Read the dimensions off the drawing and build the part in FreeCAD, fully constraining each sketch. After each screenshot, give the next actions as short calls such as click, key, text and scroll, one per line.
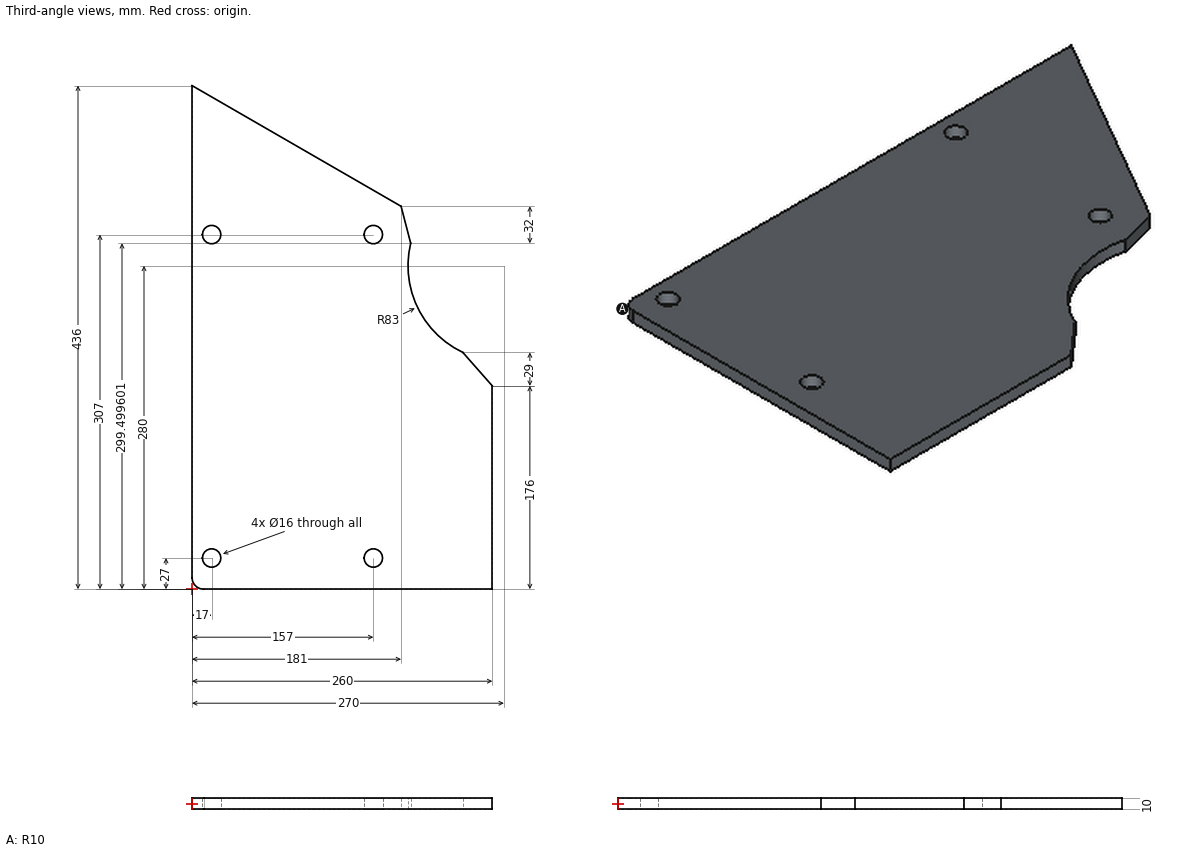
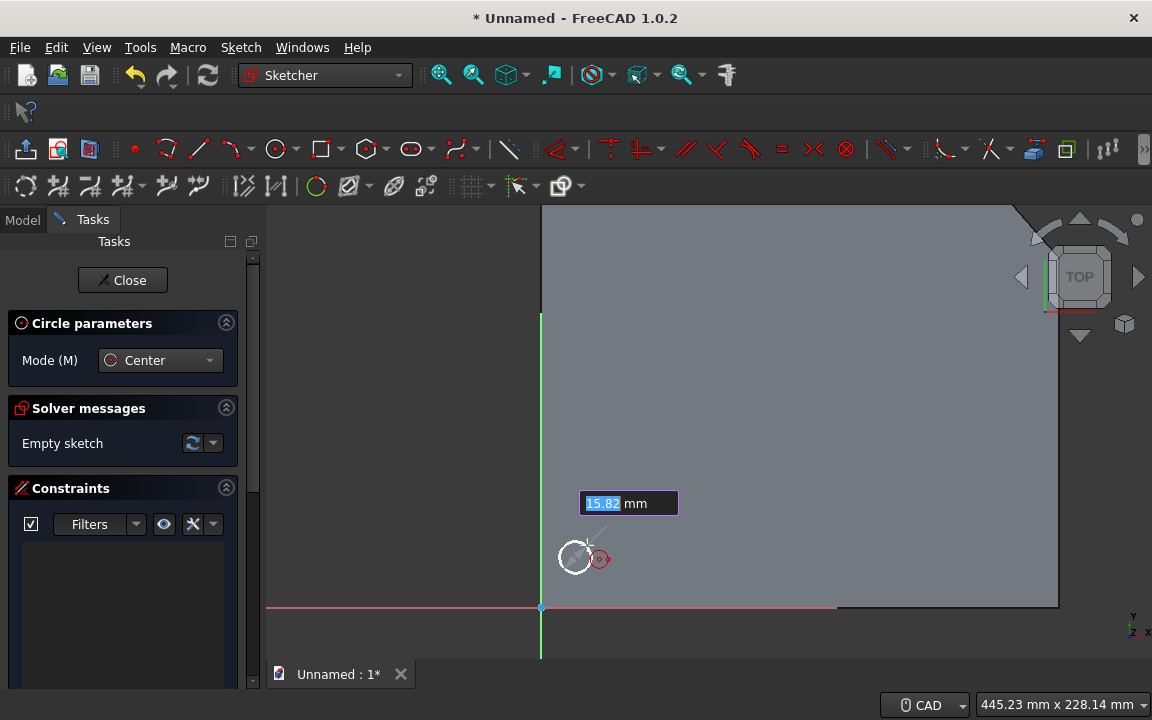
click(587, 543)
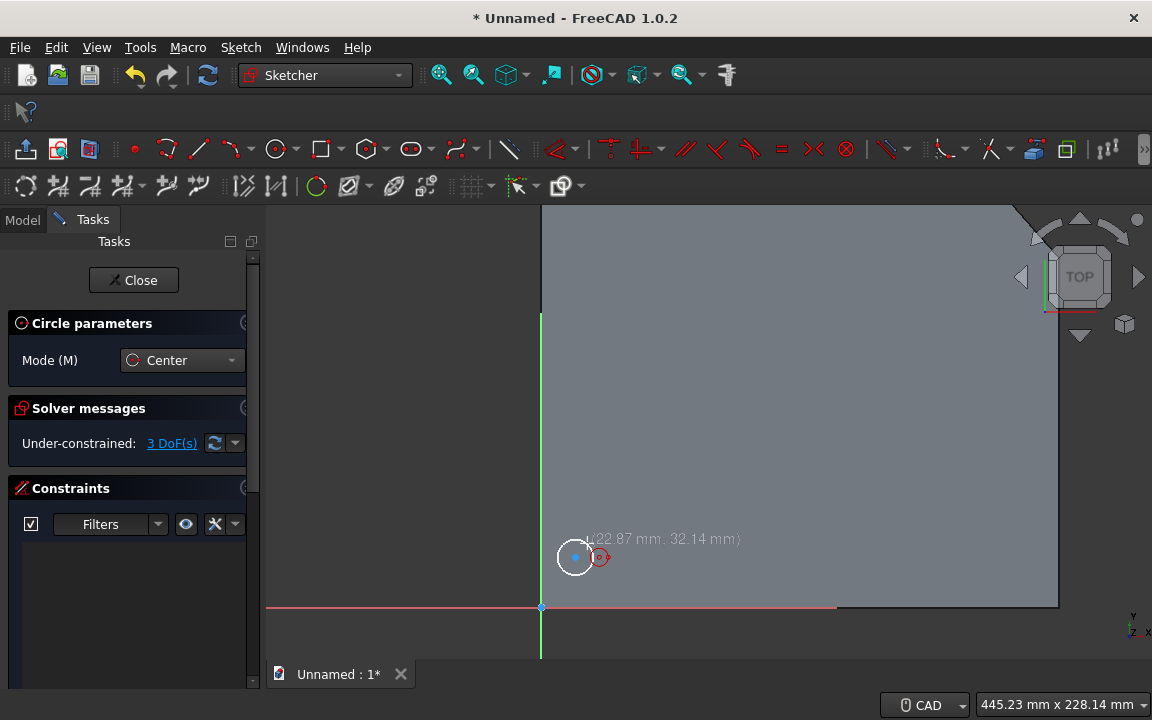
scroll(854, 554, up, 2)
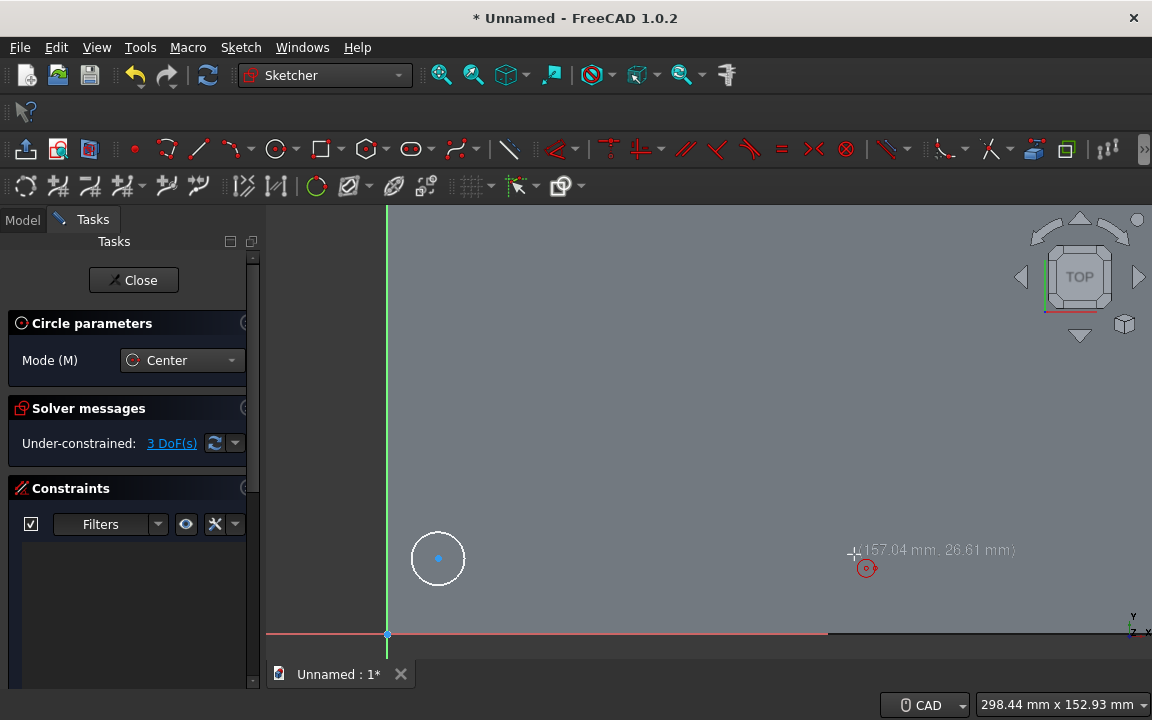
scroll(644, 546, down, 6)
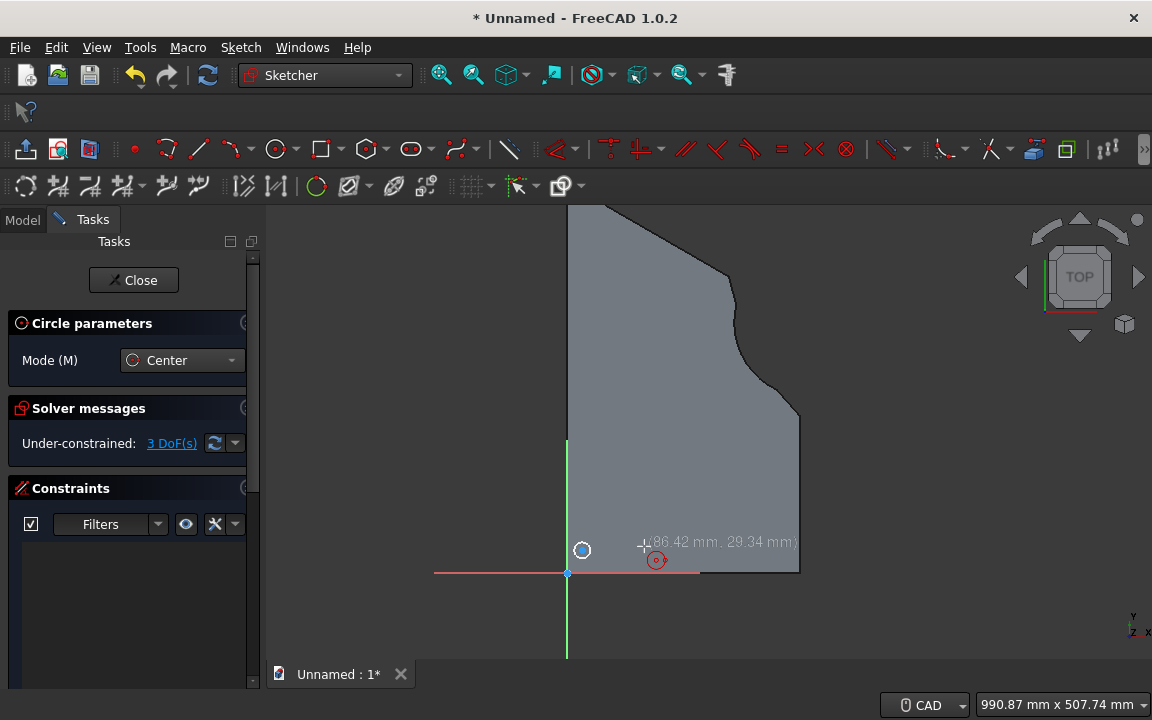
click(707, 549)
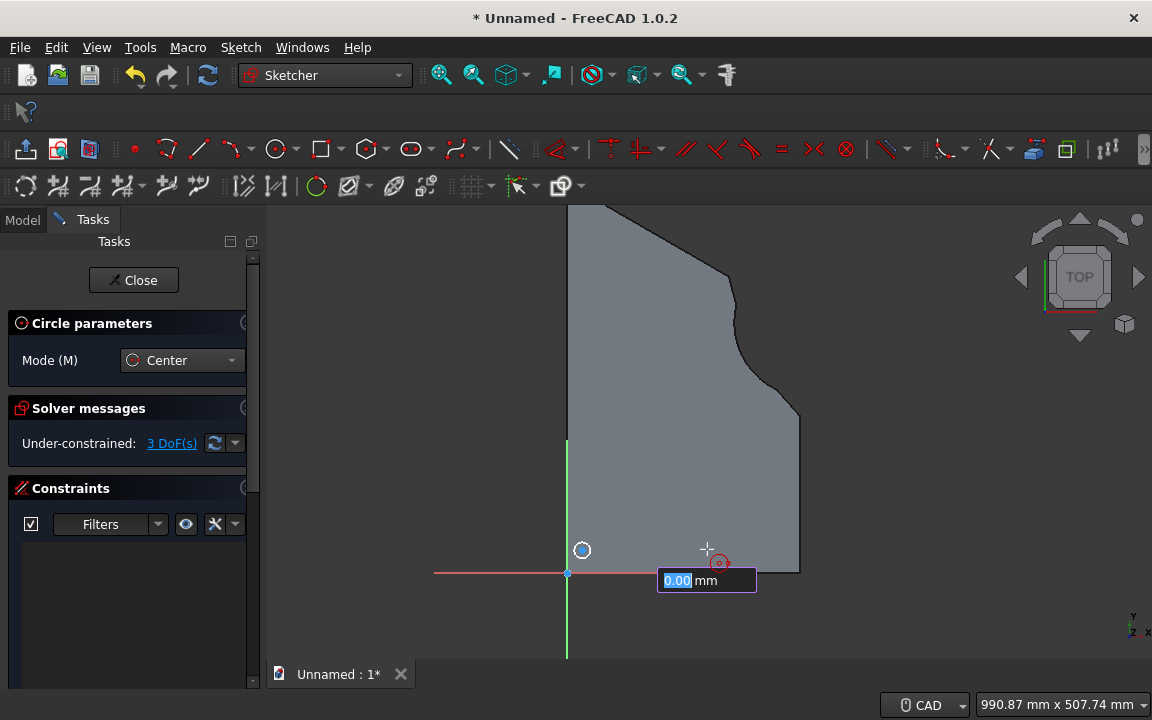
scroll(712, 544, up, 4)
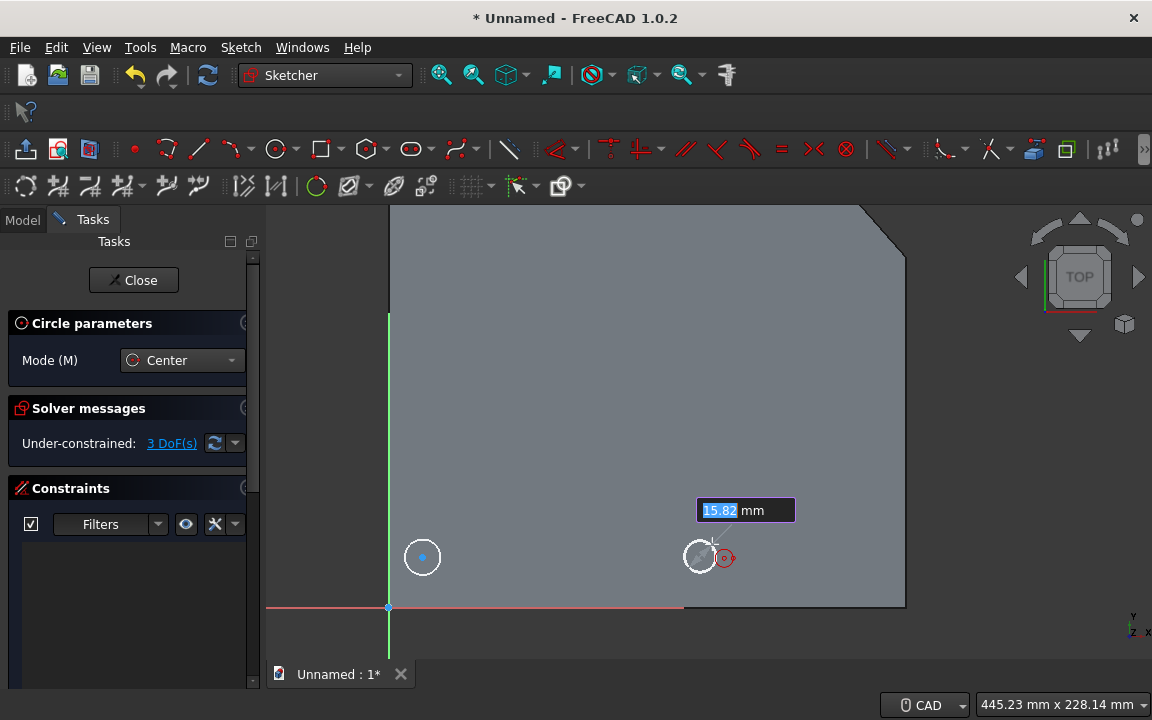
click(712, 543)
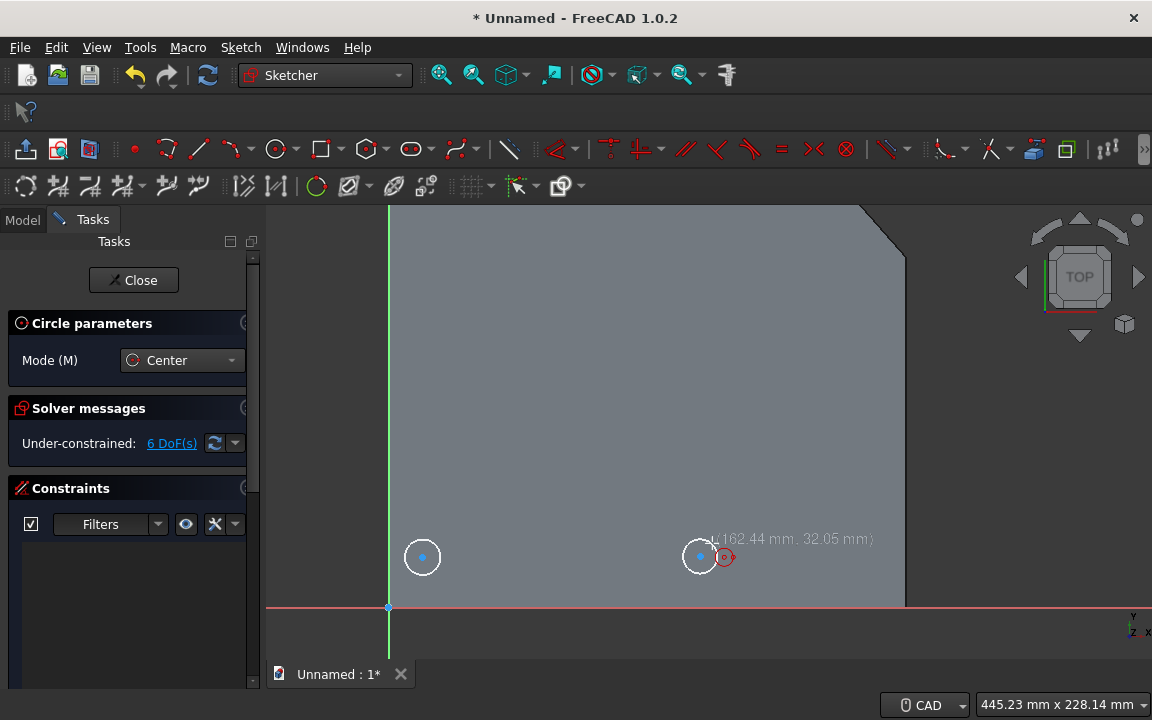
scroll(712, 544, down, 4)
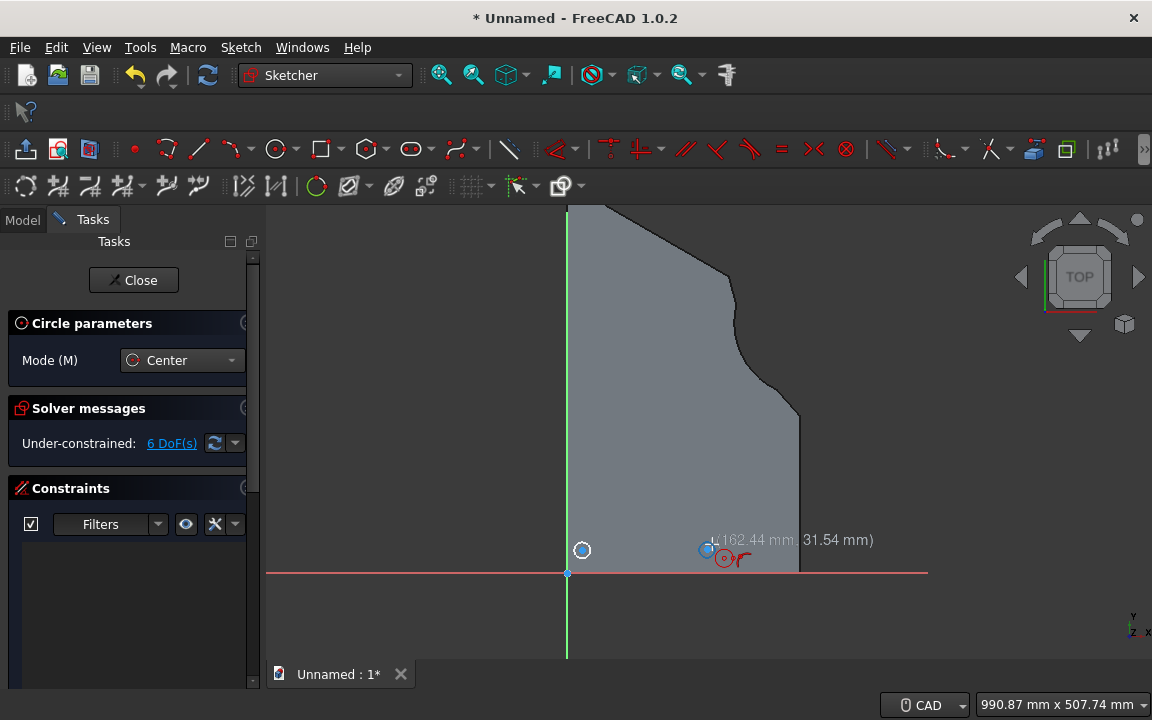
scroll(707, 299, up, 6)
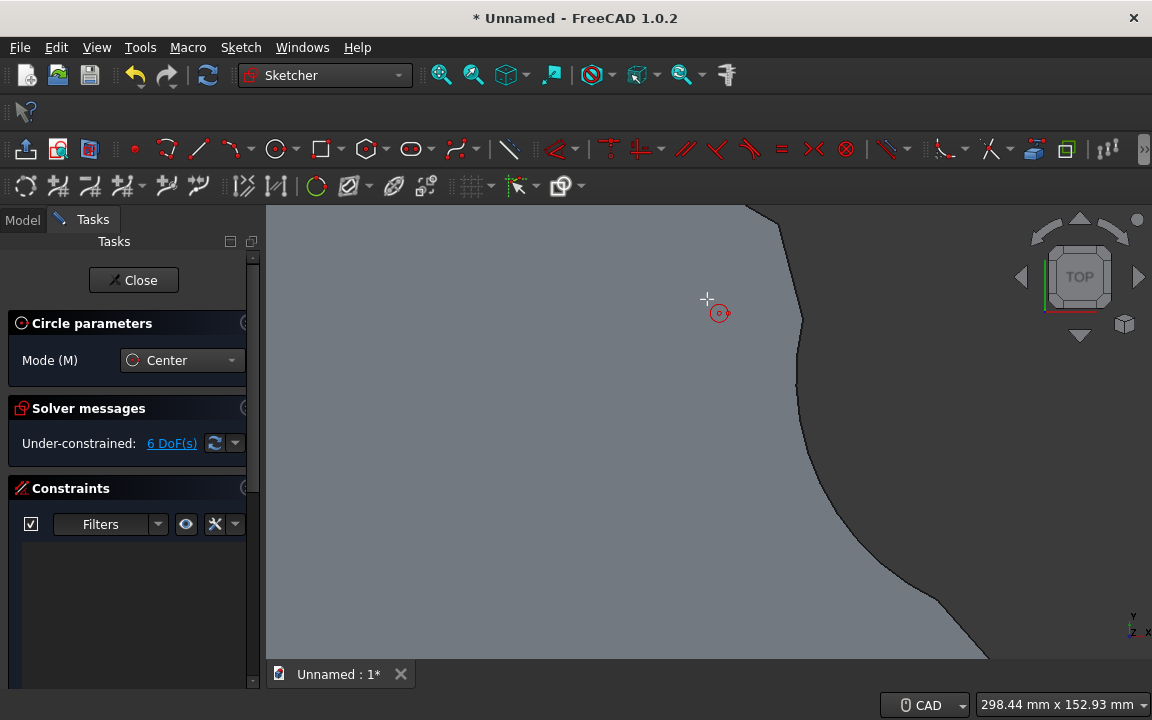
scroll(707, 299, down, 6)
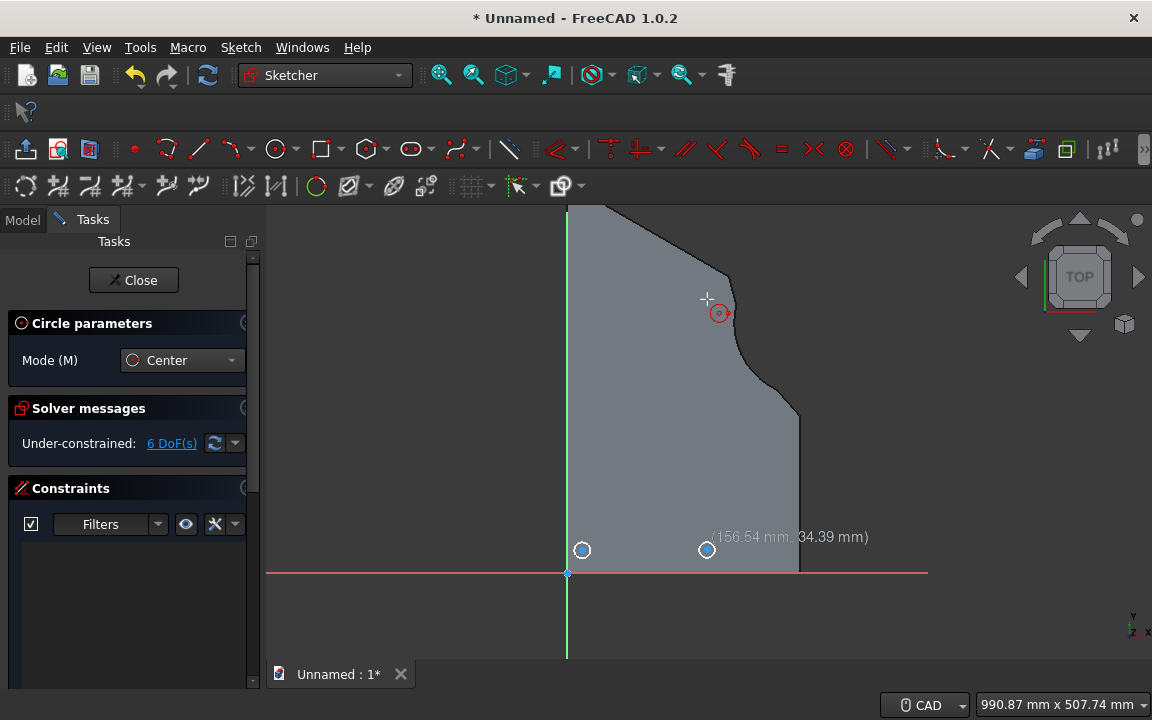
click(707, 299)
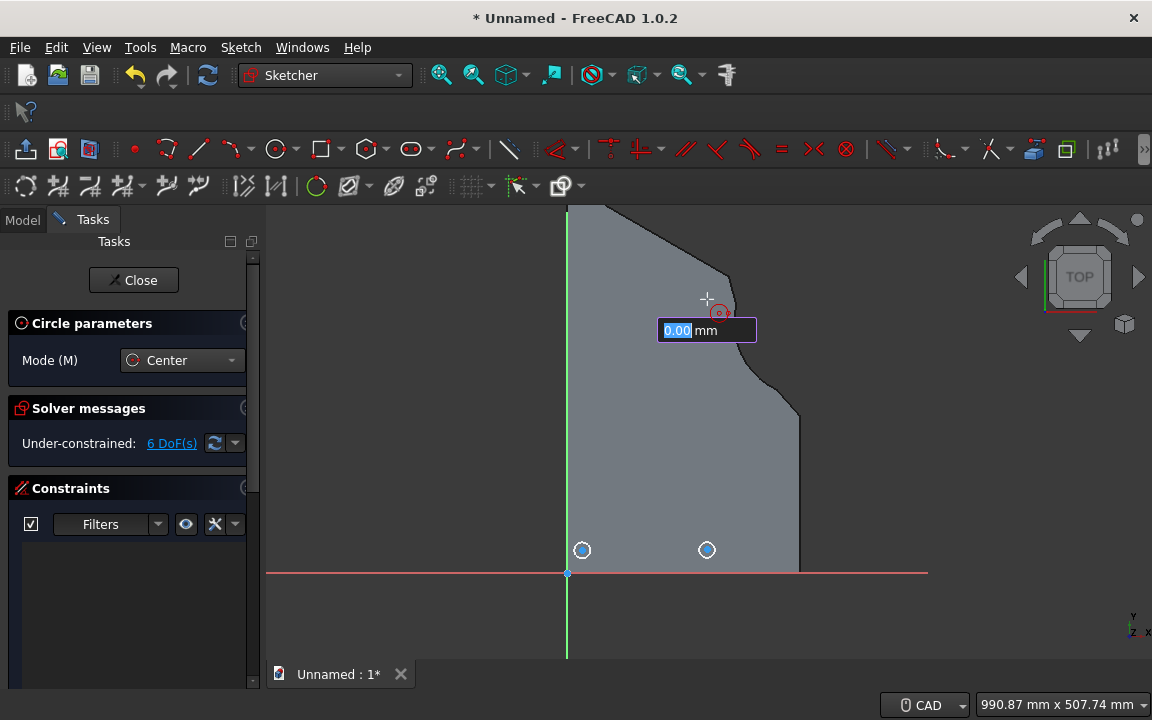
scroll(712, 293, up, 4)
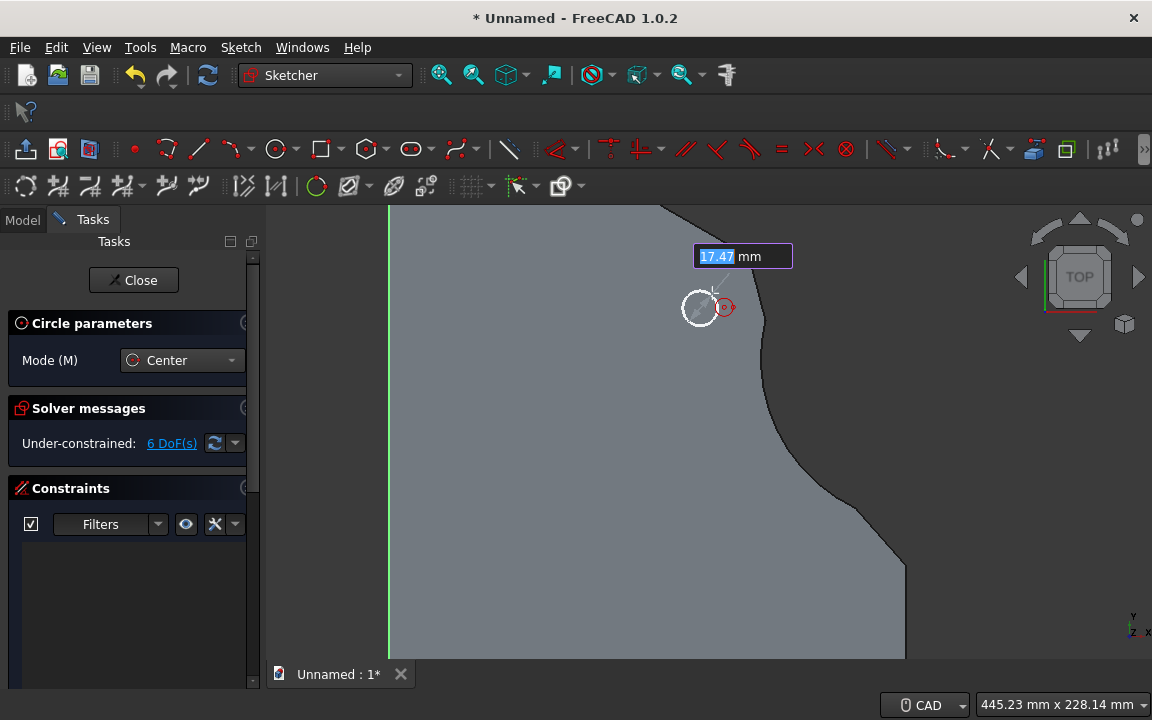
click(712, 294)